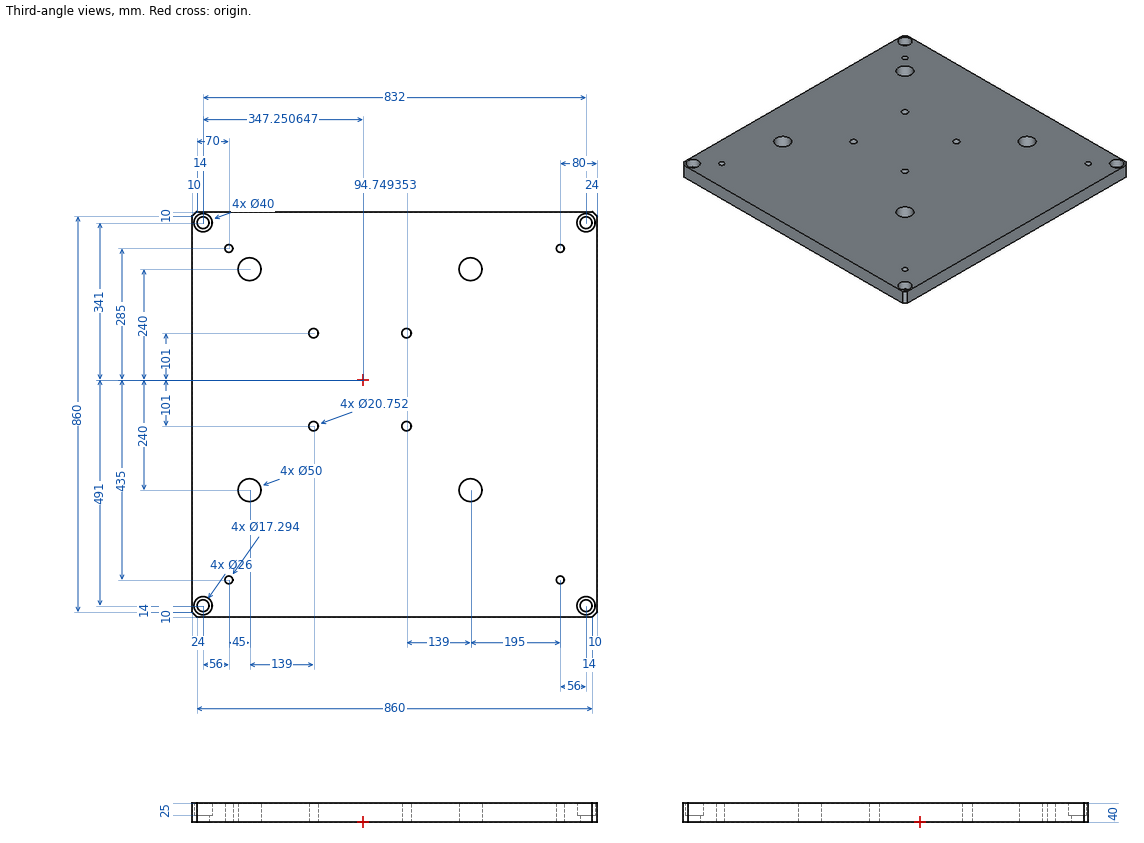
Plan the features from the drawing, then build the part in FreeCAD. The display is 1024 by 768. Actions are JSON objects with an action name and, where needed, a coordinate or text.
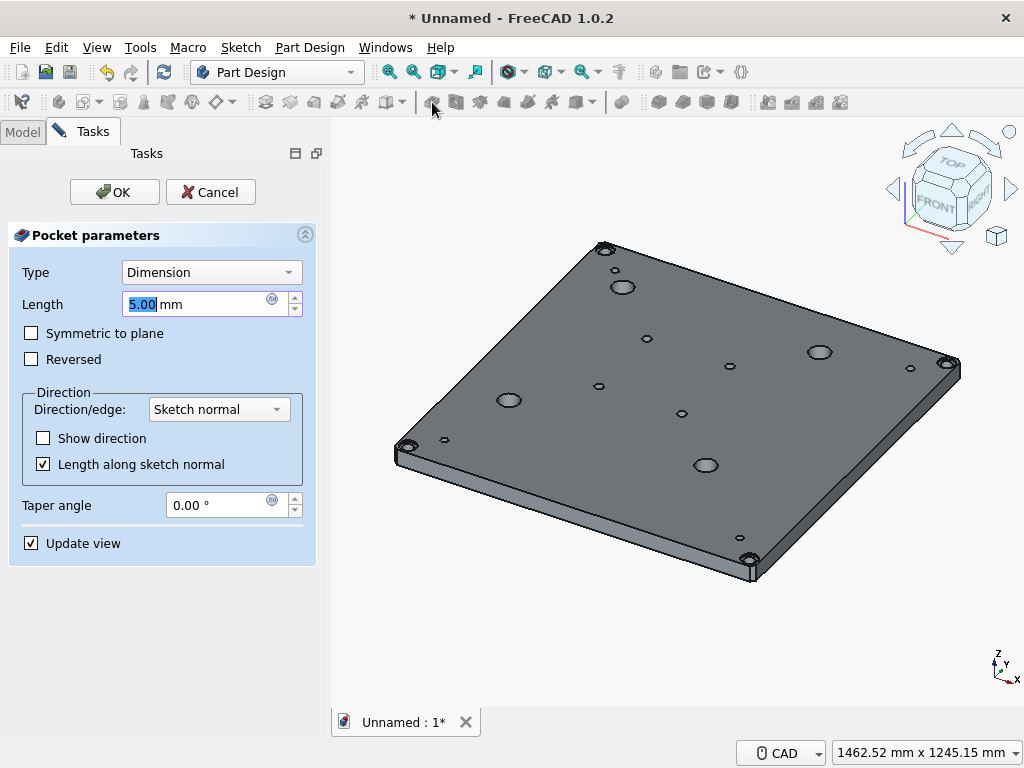
{"action": "type", "text": "25"}
{"action": "key", "text": "Tab"}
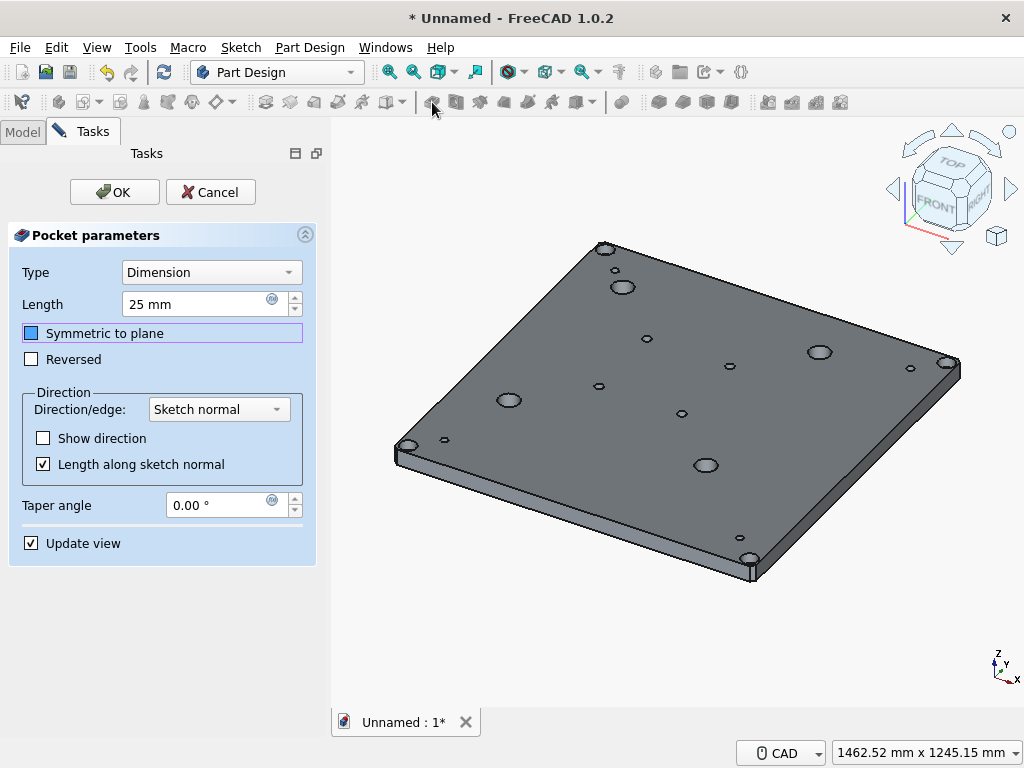
{"action": "left_click", "coordinate": [115, 192]}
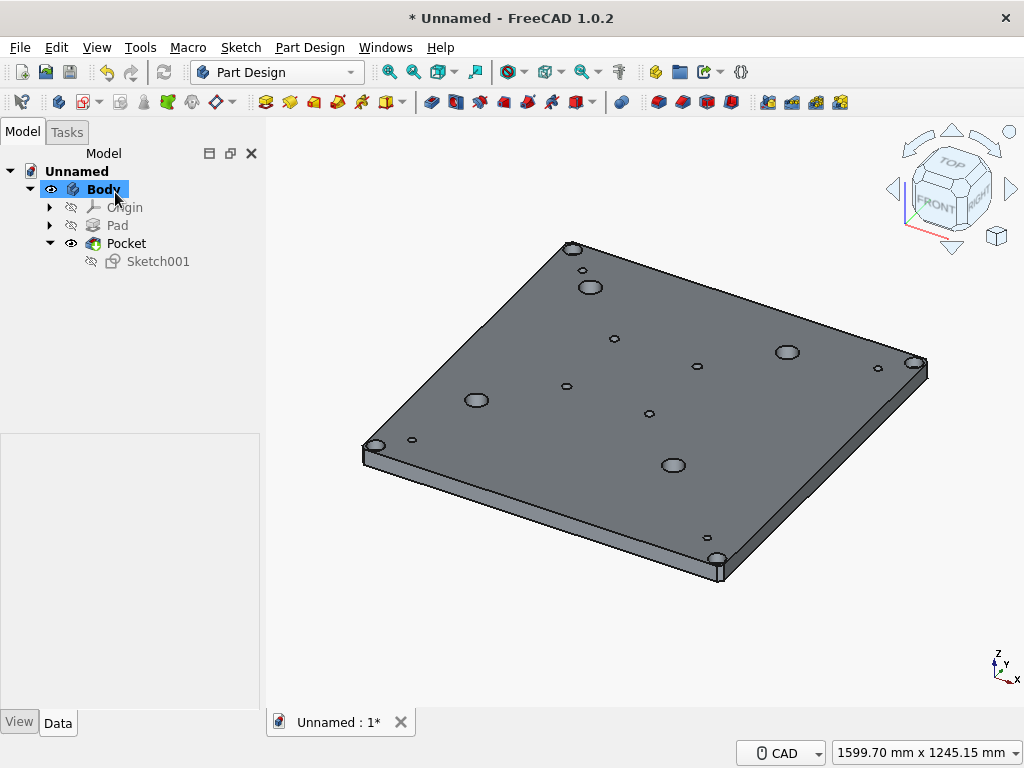
{"action": "key", "text": "0"}